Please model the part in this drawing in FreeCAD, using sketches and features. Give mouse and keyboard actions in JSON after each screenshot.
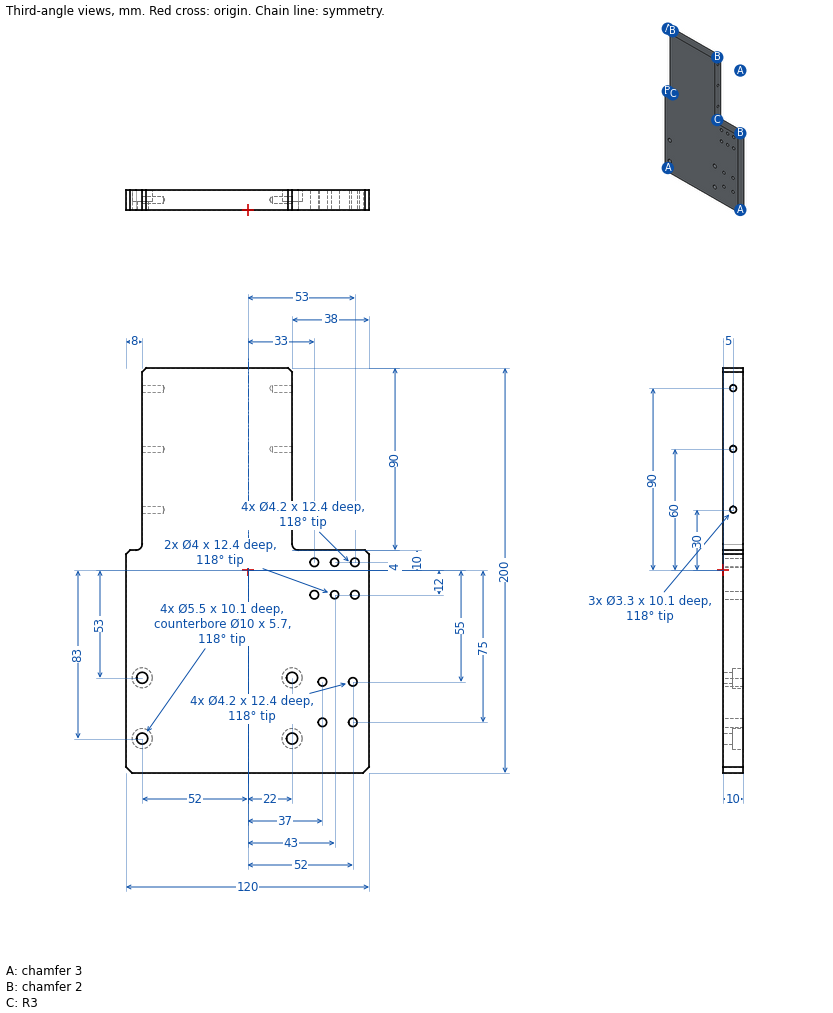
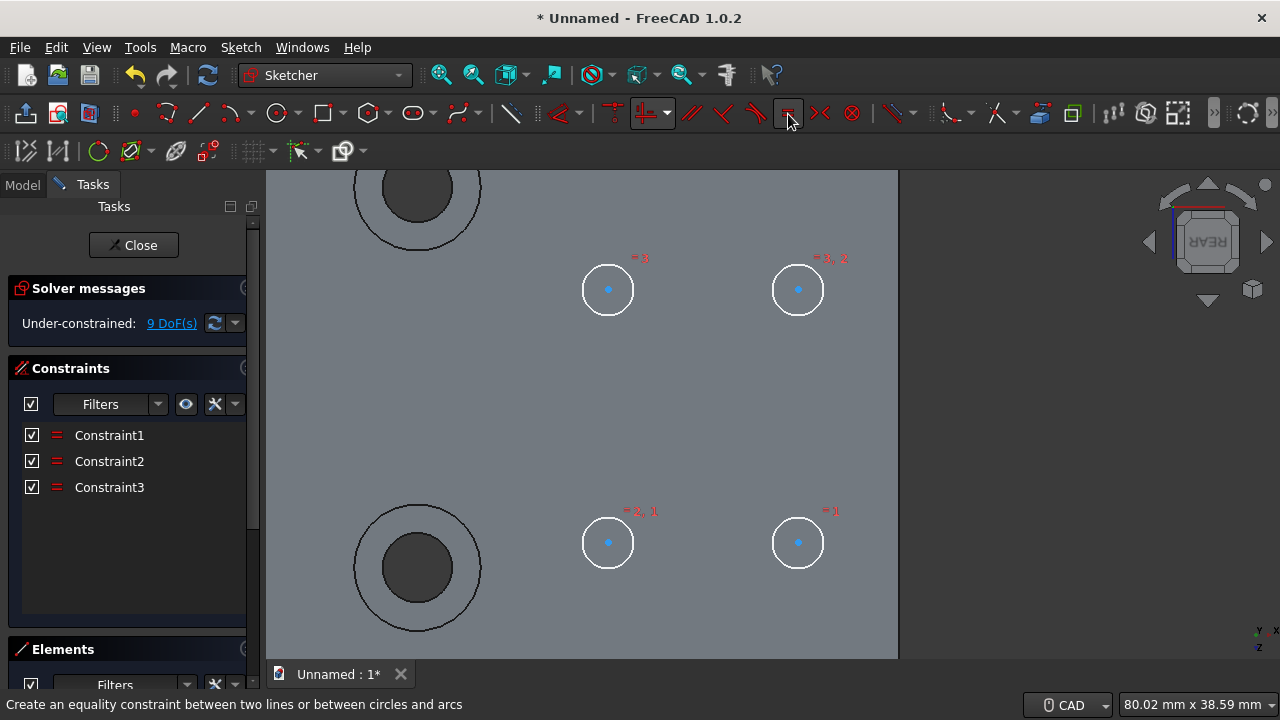
{"action": "left_click", "coordinate": [798, 543]}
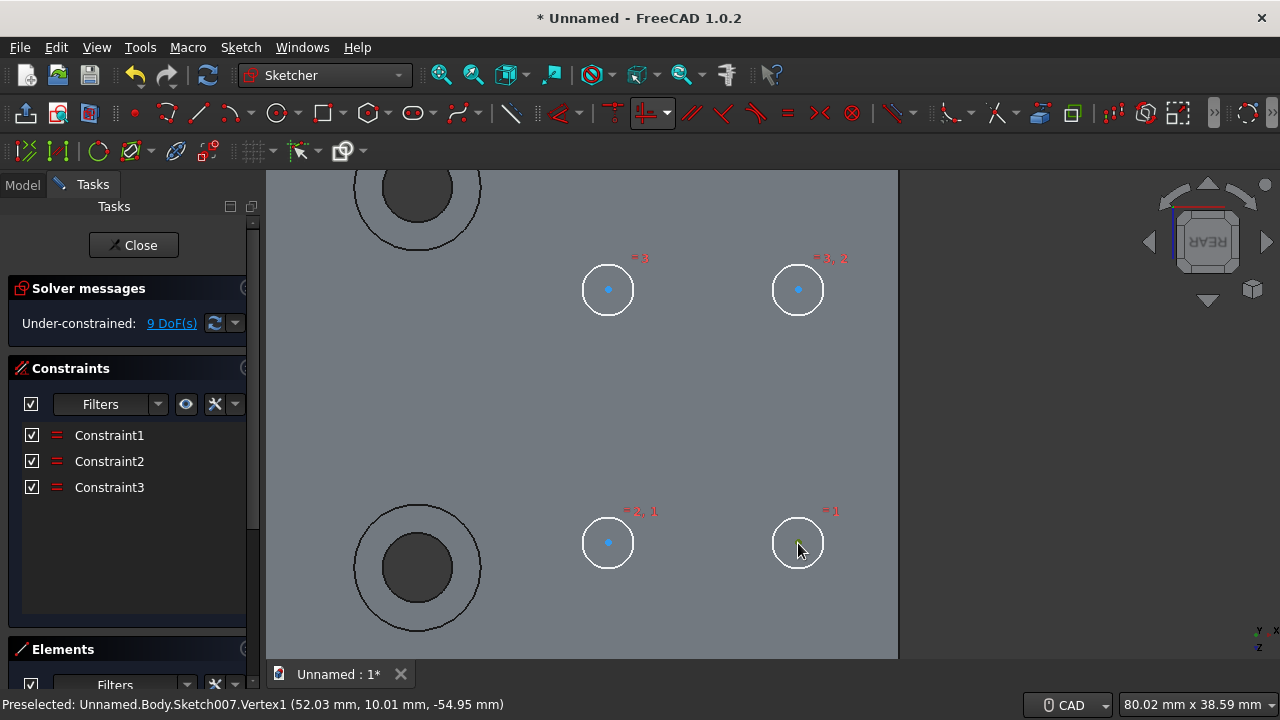
{"action": "left_click", "coordinate": [608, 543]}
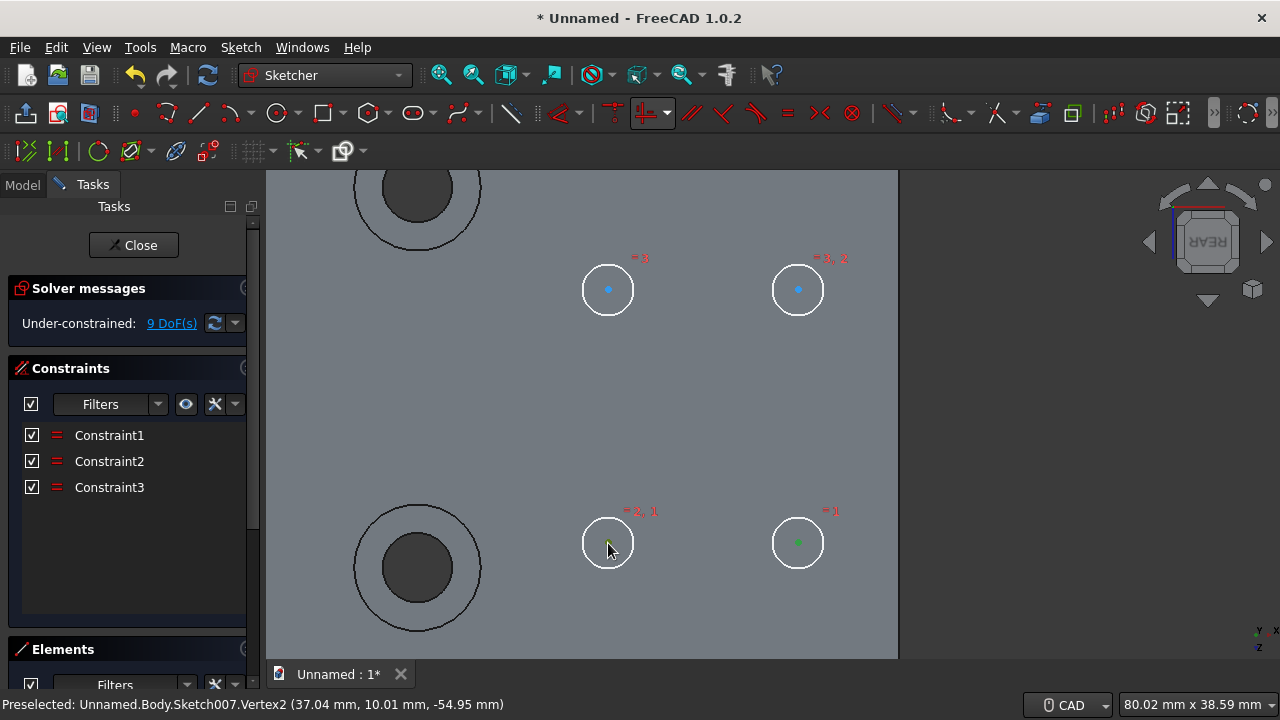
{"action": "left_click", "coordinate": [670, 114]}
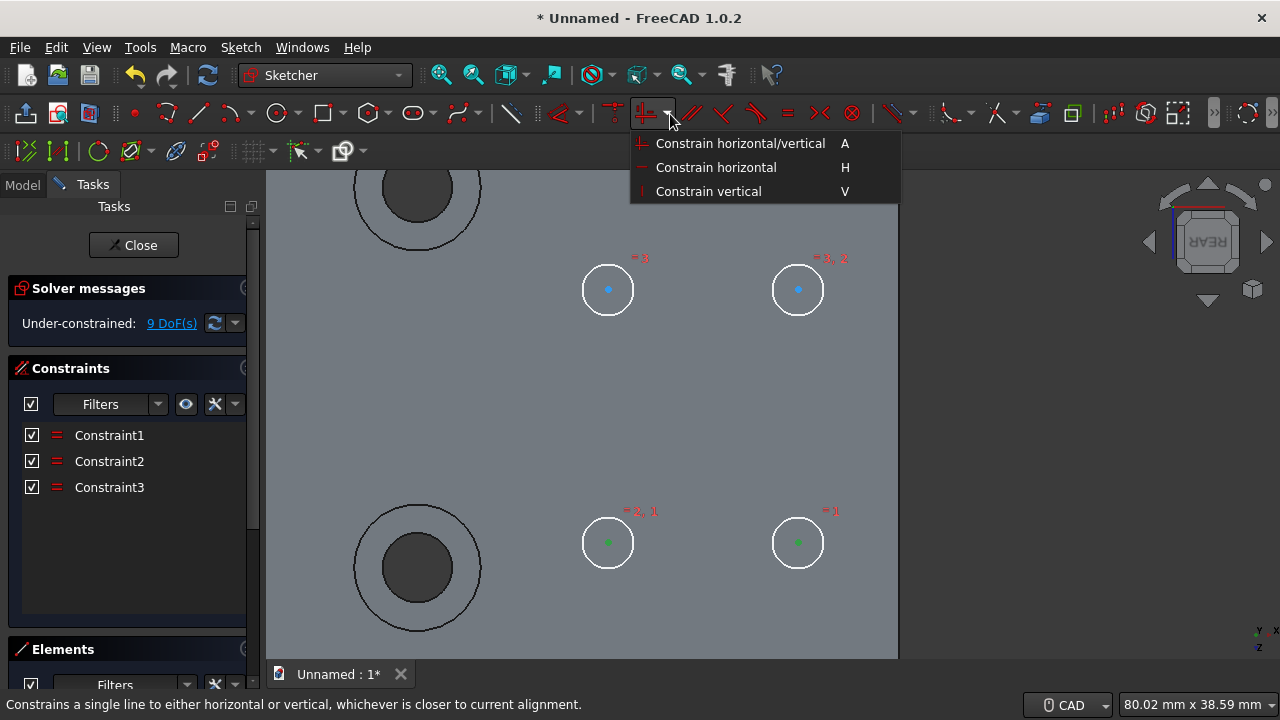
{"action": "left_click", "coordinate": [766, 167]}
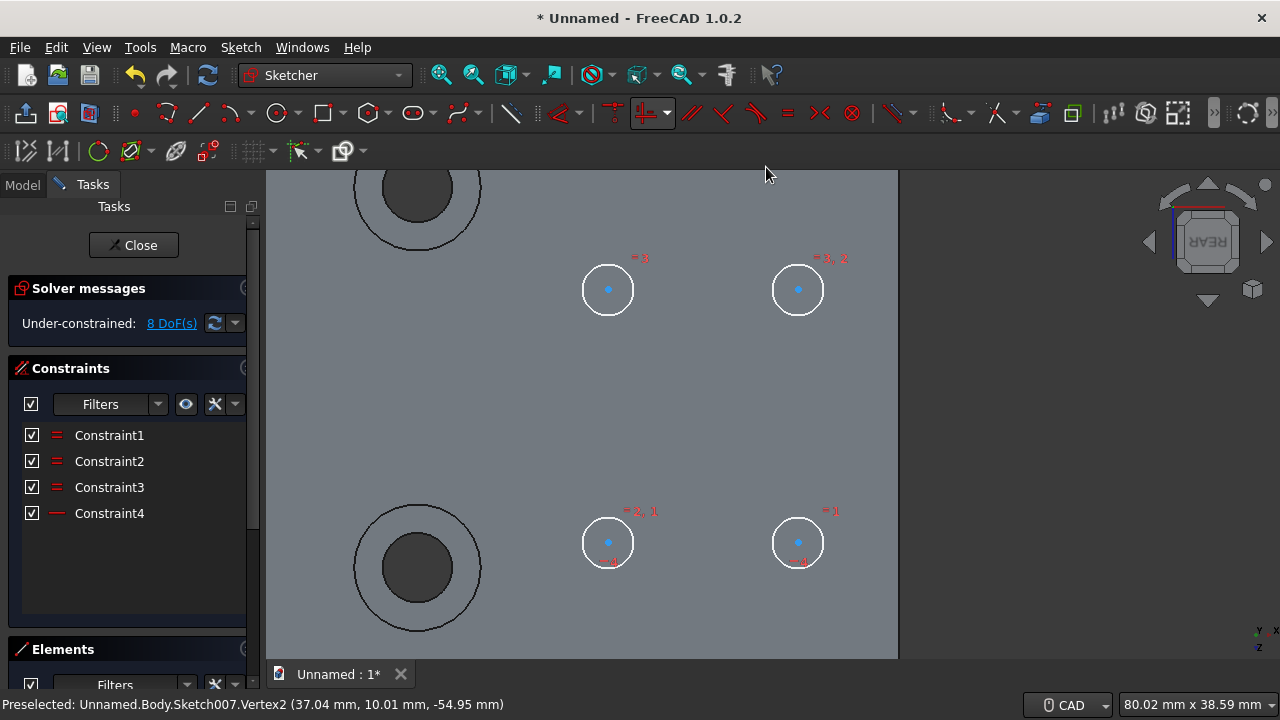
{"action": "left_click", "coordinate": [798, 543]}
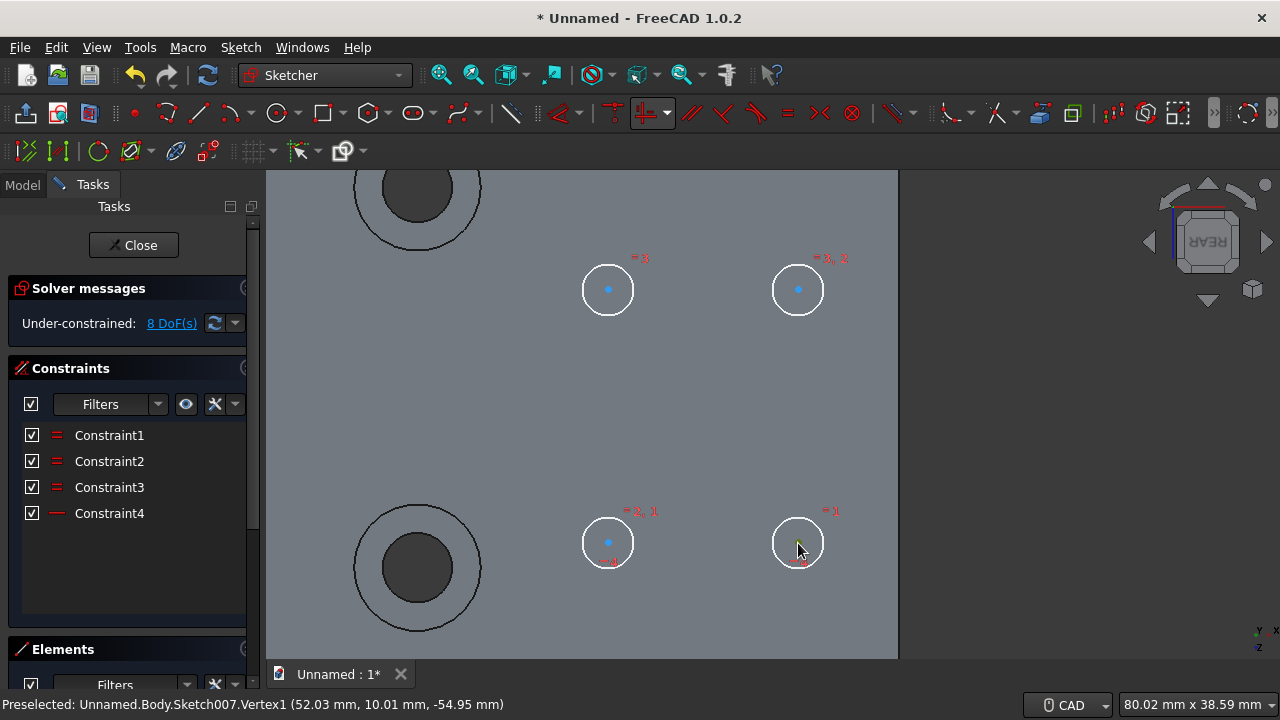
{"action": "left_click", "coordinate": [798, 290]}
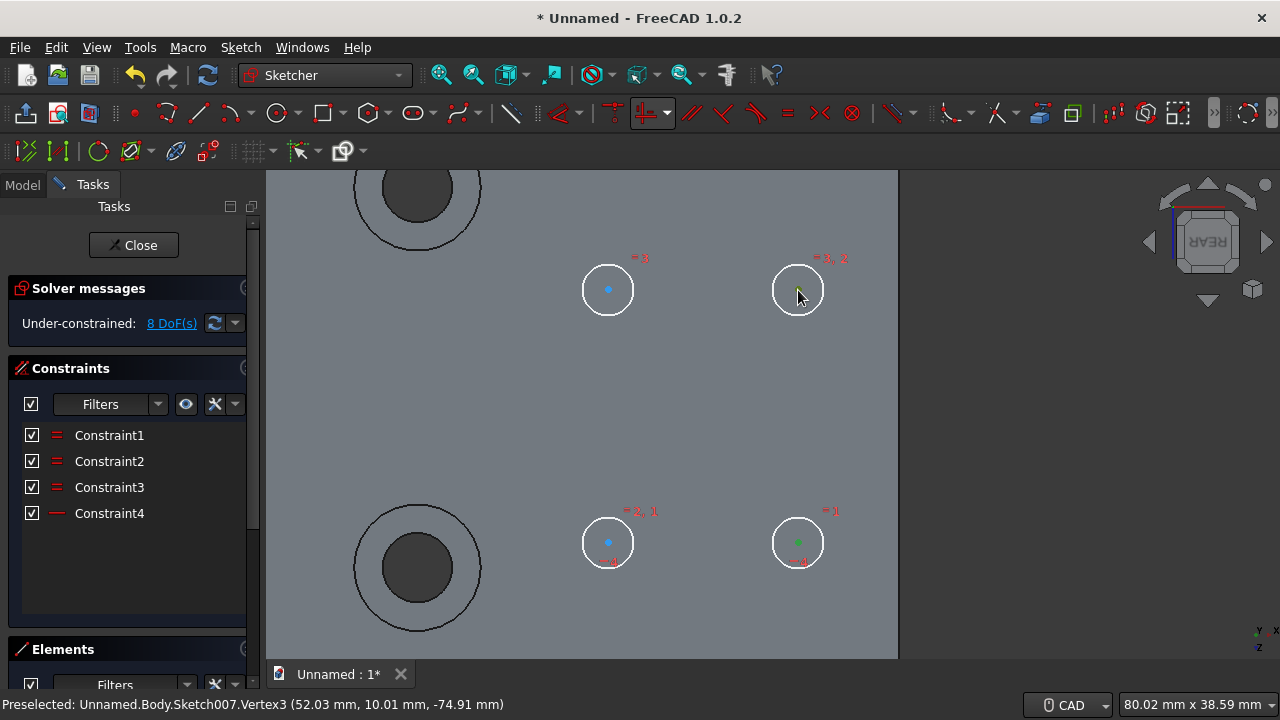
{"action": "left_click", "coordinate": [670, 114]}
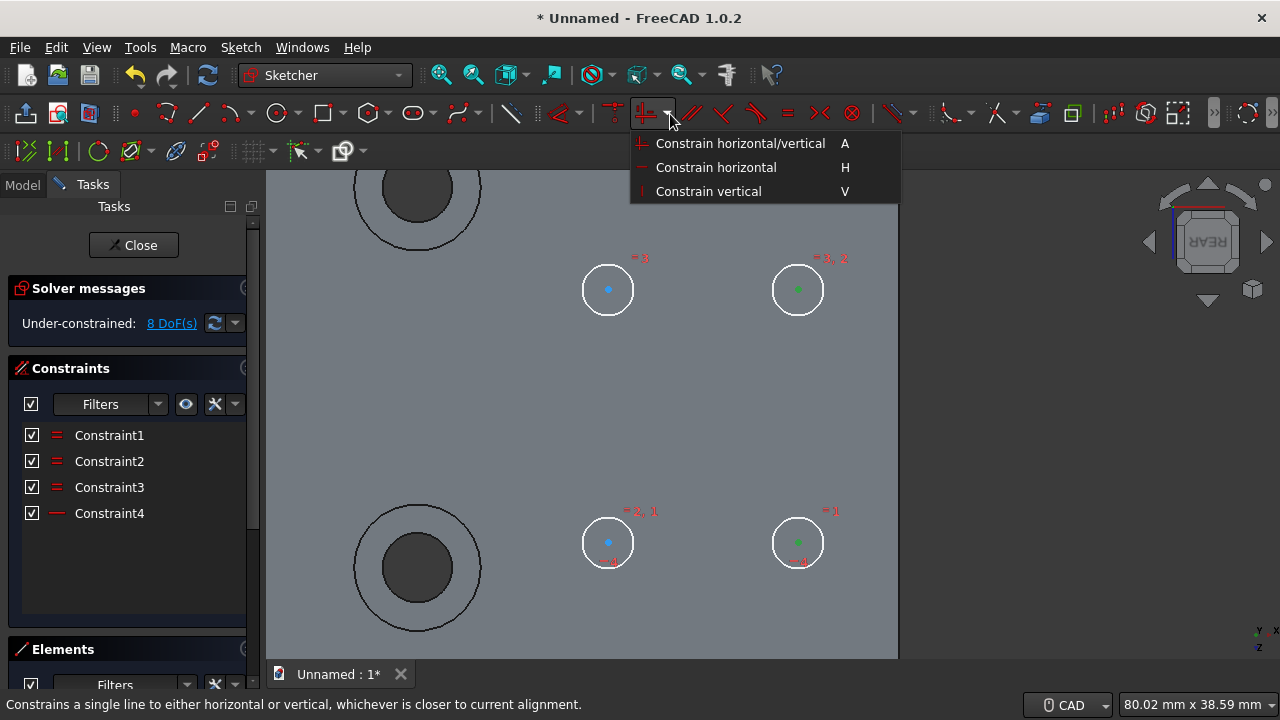
{"action": "left_click", "coordinate": [766, 191]}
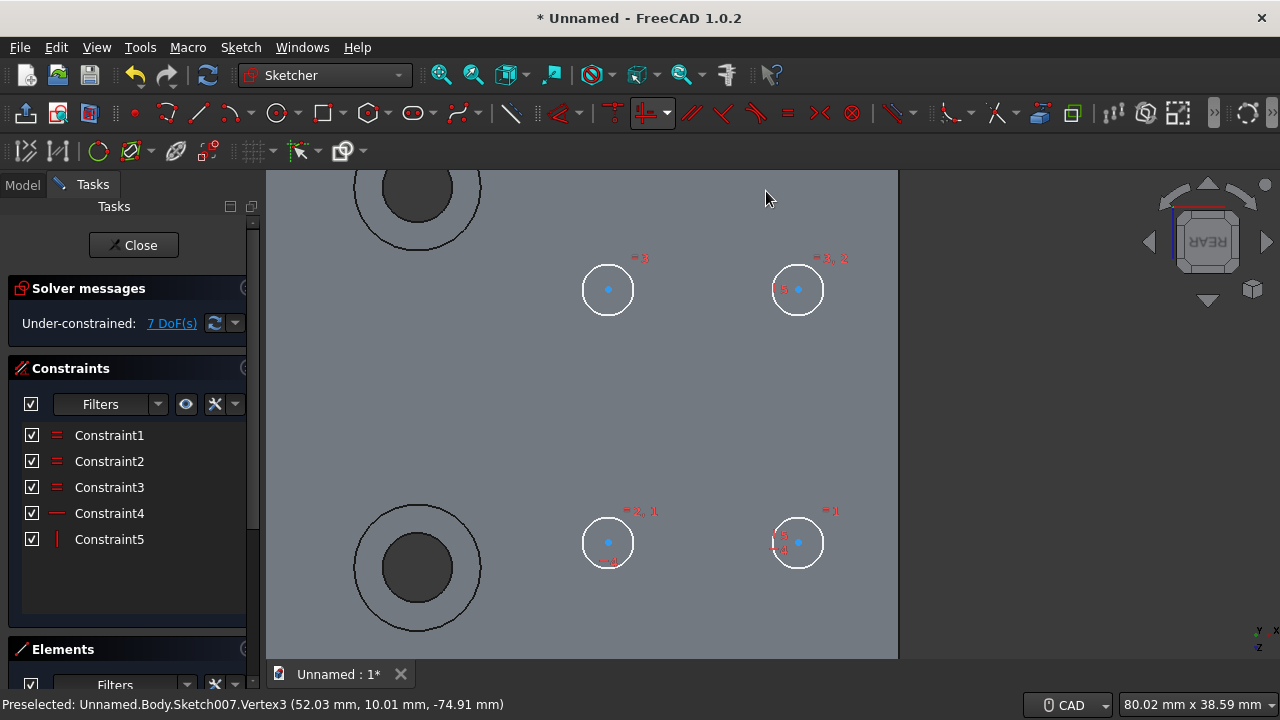
{"action": "left_click", "coordinate": [608, 543]}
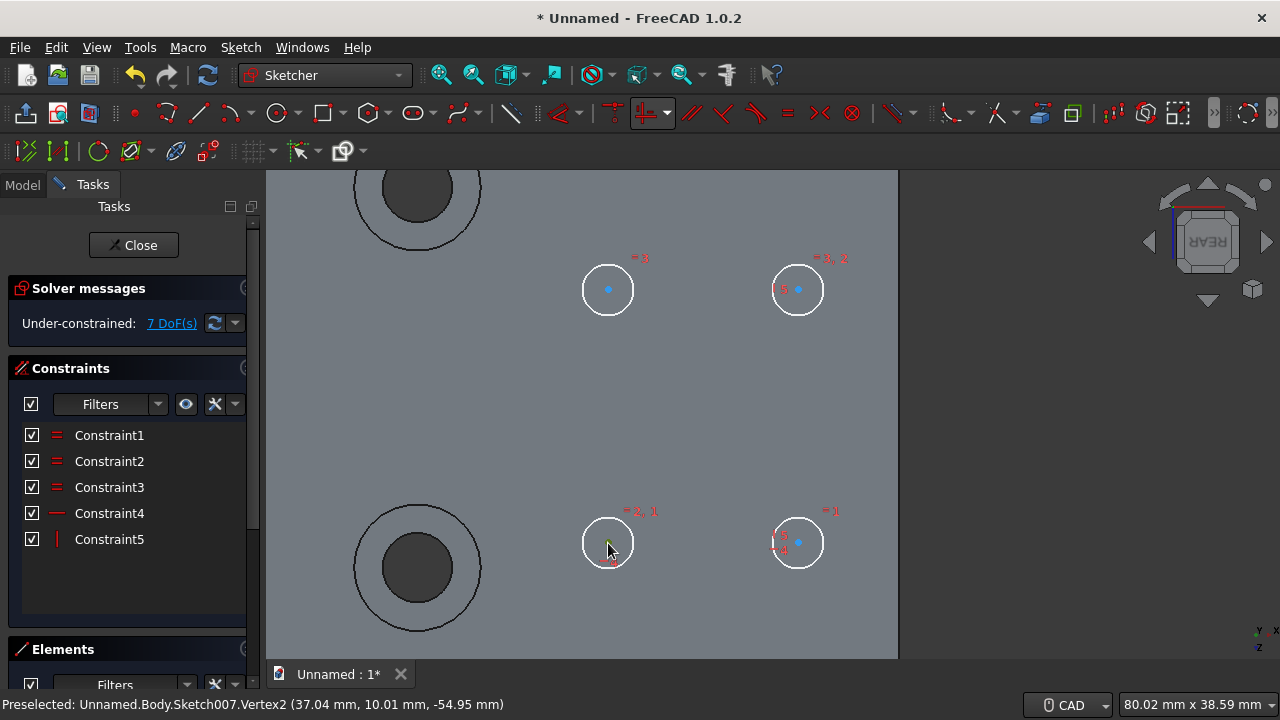
{"action": "left_click", "coordinate": [608, 290]}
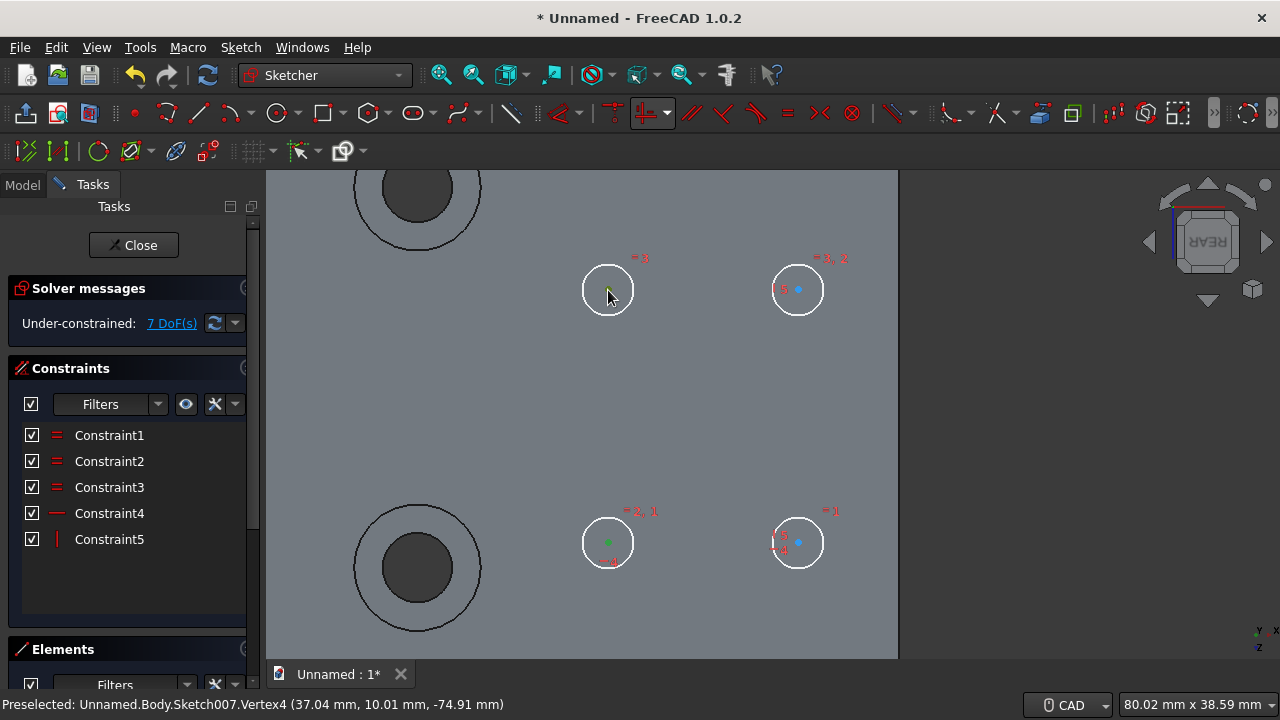
{"action": "left_click", "coordinate": [670, 114]}